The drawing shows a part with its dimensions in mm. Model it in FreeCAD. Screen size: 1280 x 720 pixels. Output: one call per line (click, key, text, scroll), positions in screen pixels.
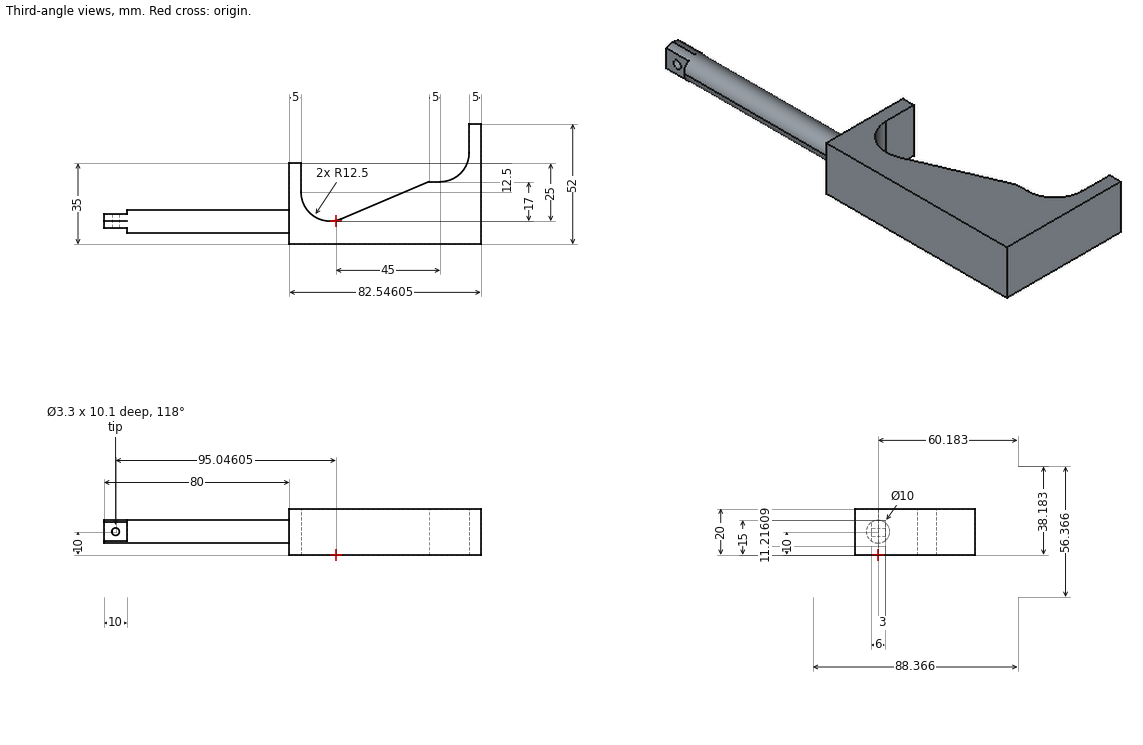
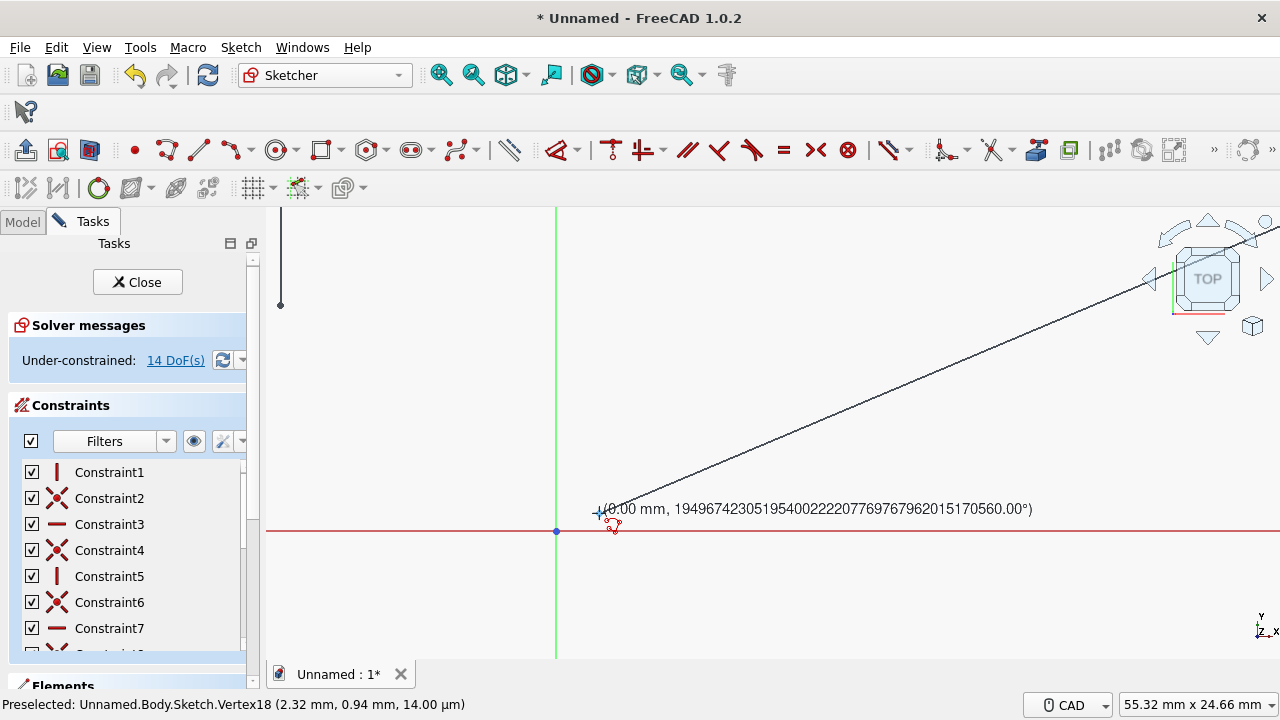
click(232, 150)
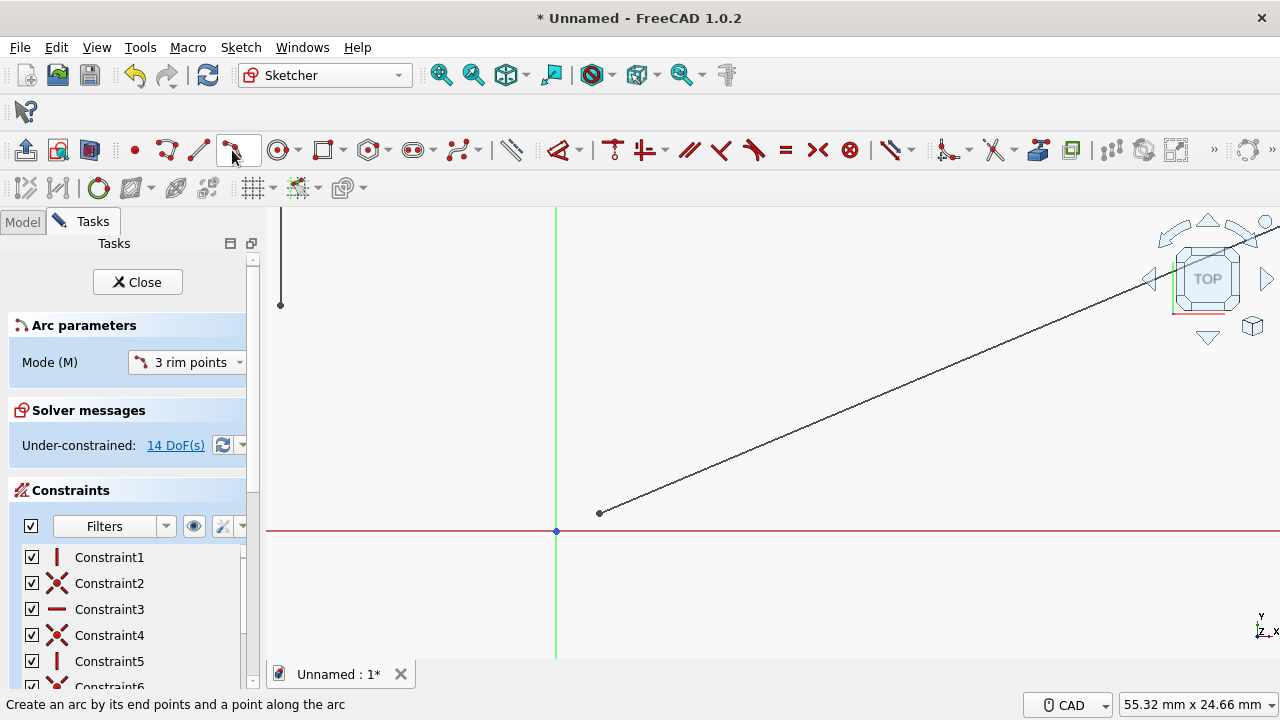
scroll(601, 517, down, 6)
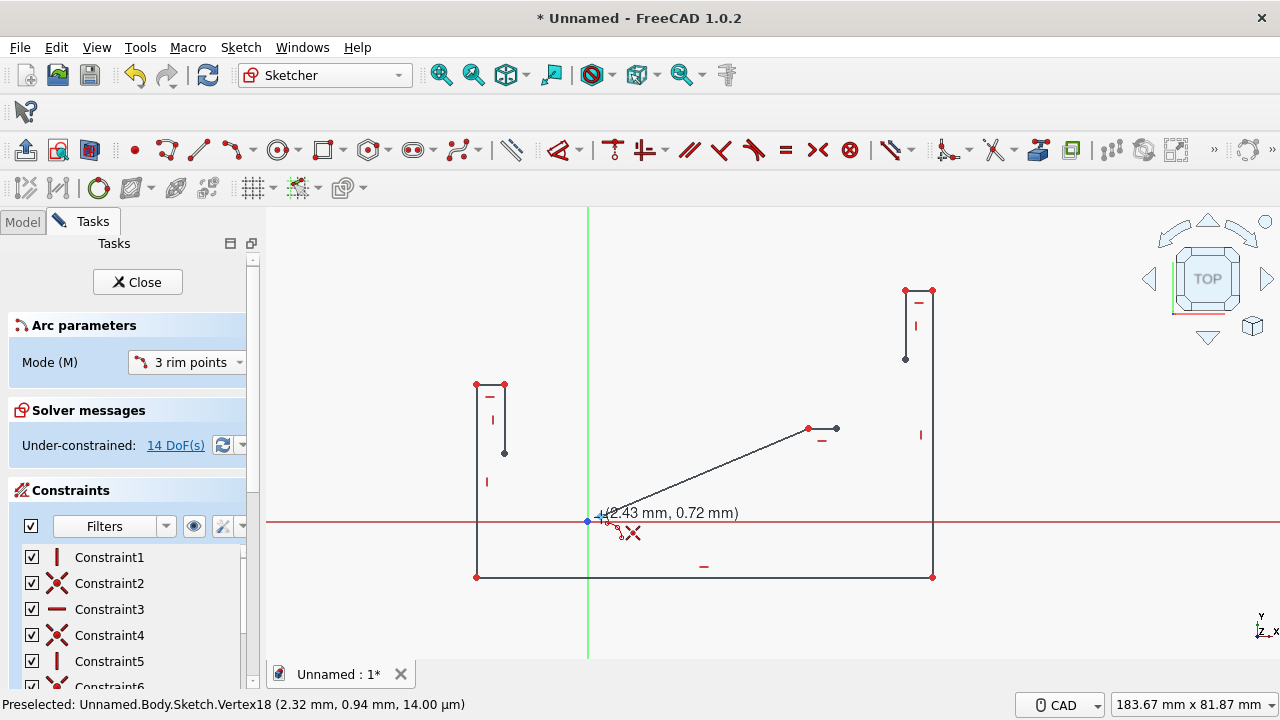
click(906, 360)
click(837, 429)
click(885, 408)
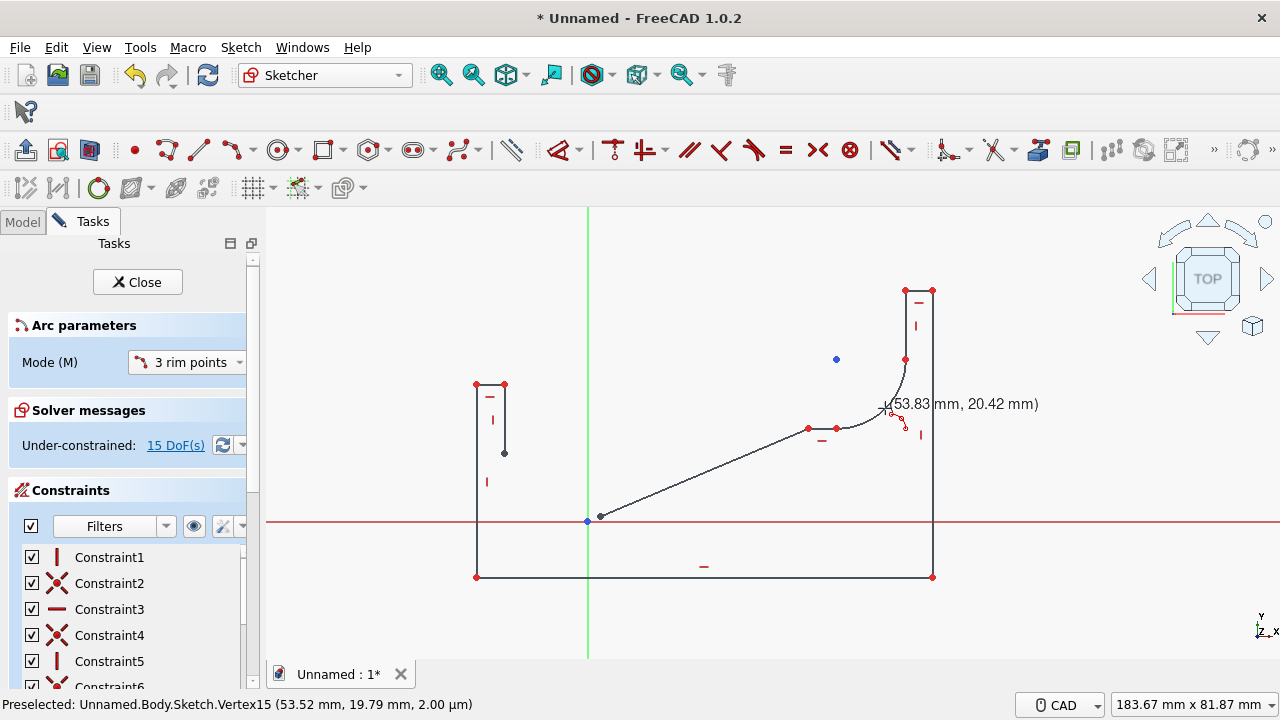
scroll(601, 516, up, 6)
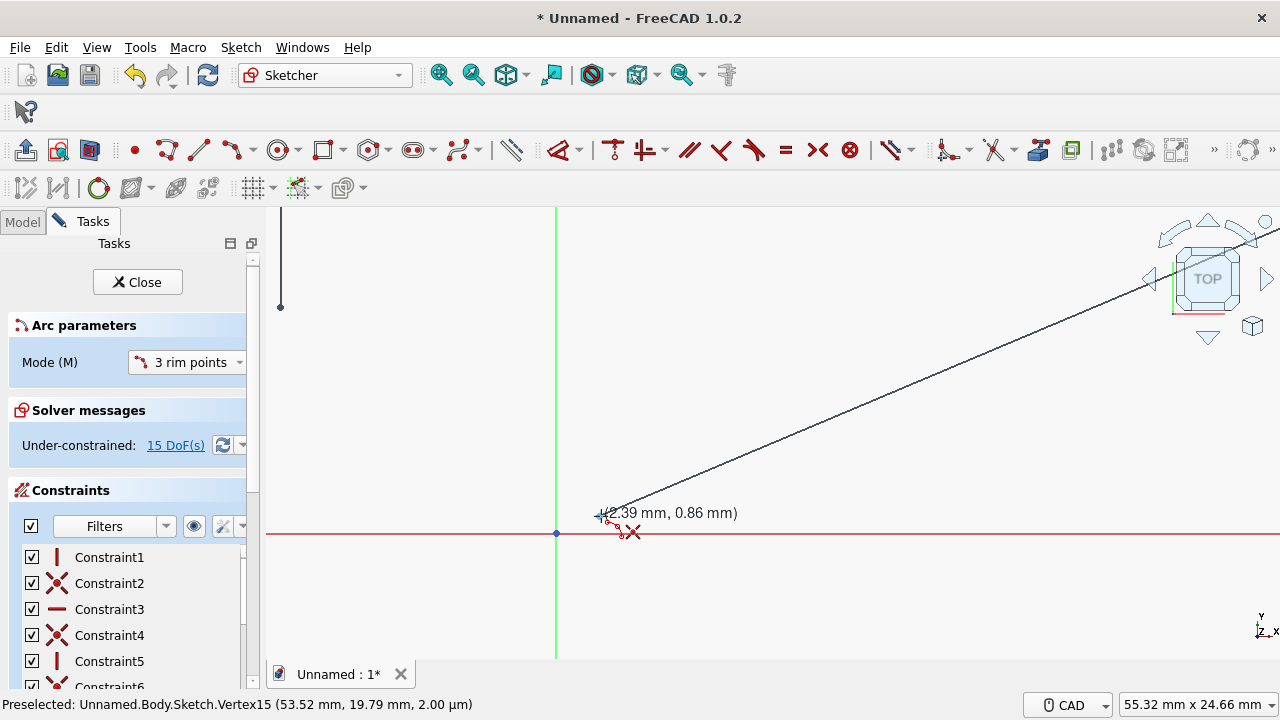
click(599, 516)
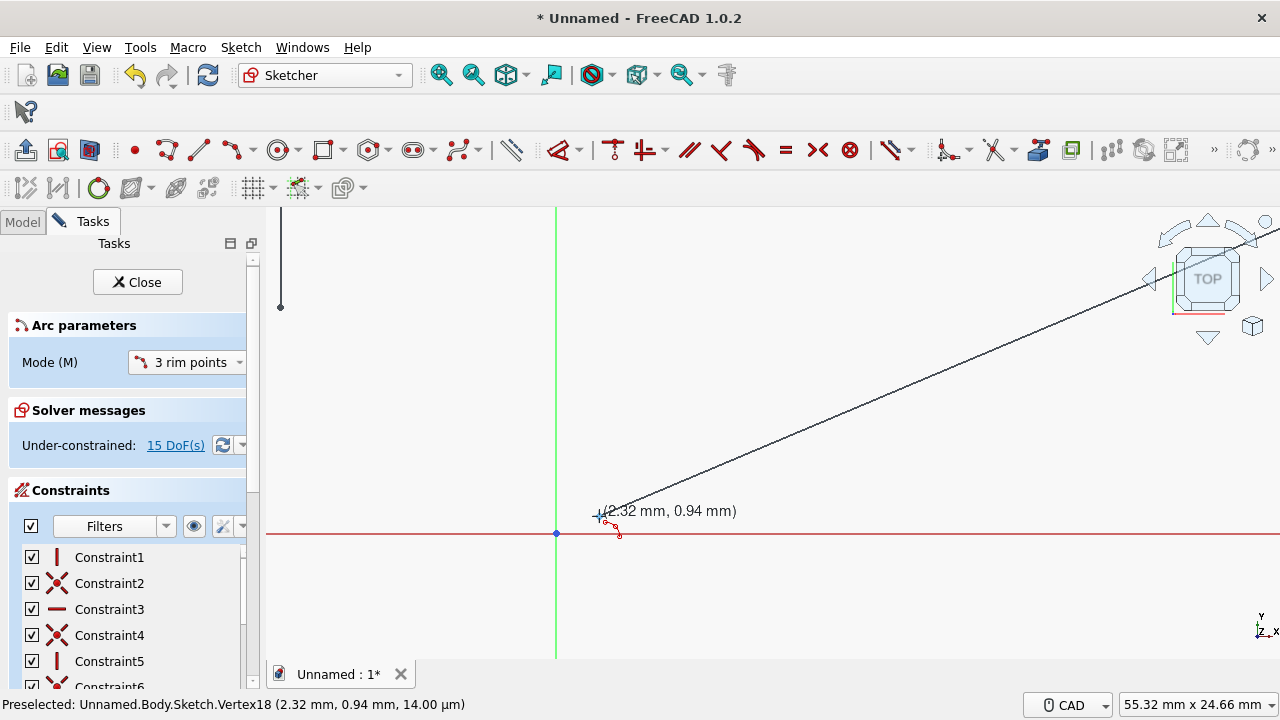
scroll(601, 516, down, 6)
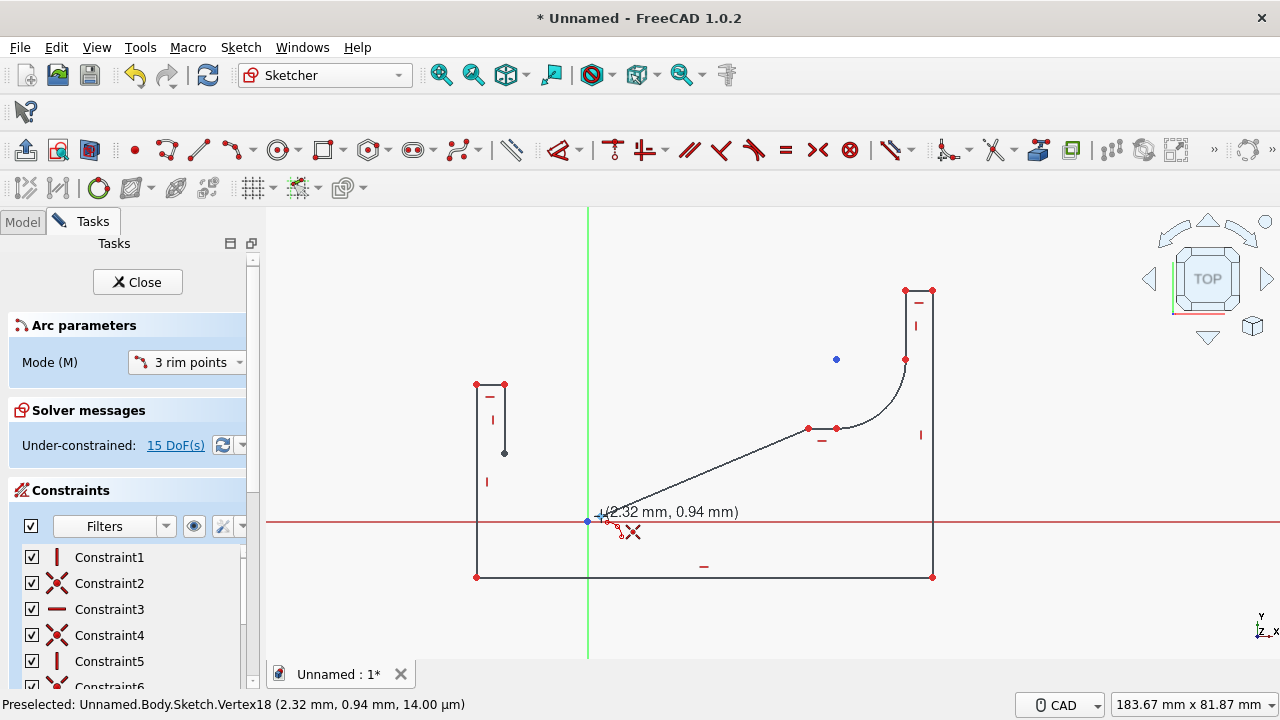
click(505, 454)
click(525, 502)
key(Escape)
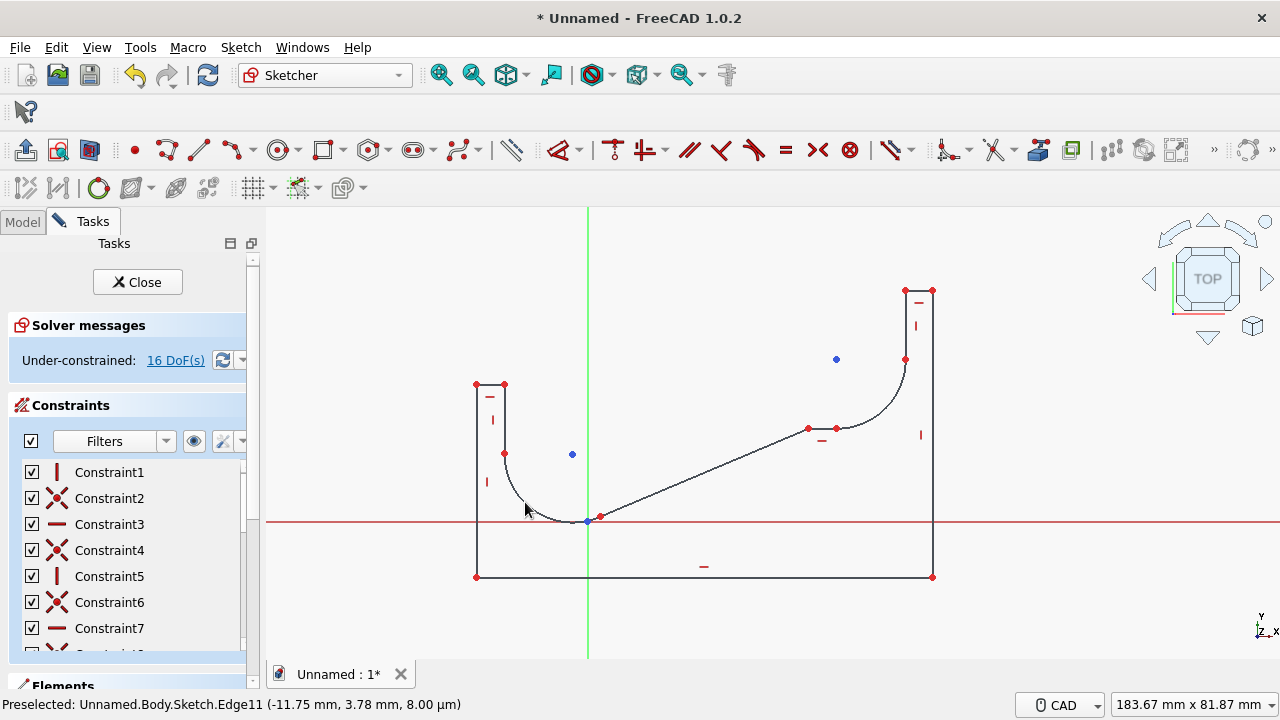
click(505, 433)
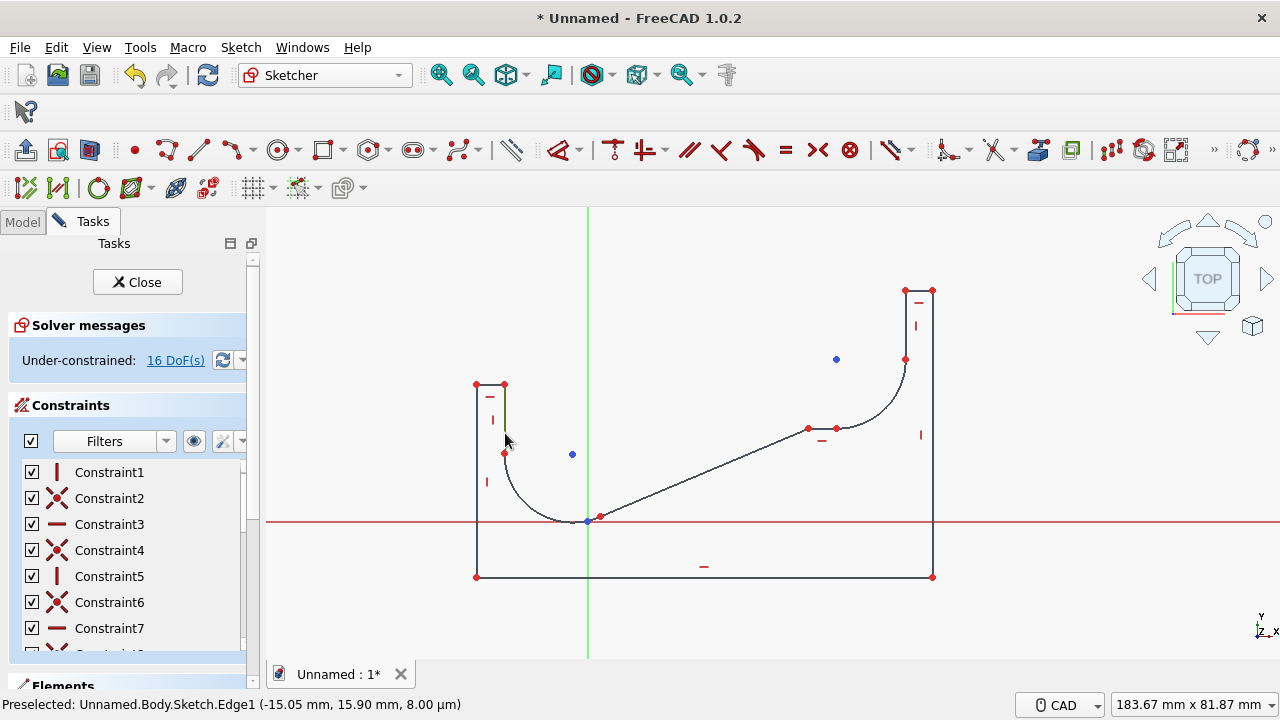
click(516, 492)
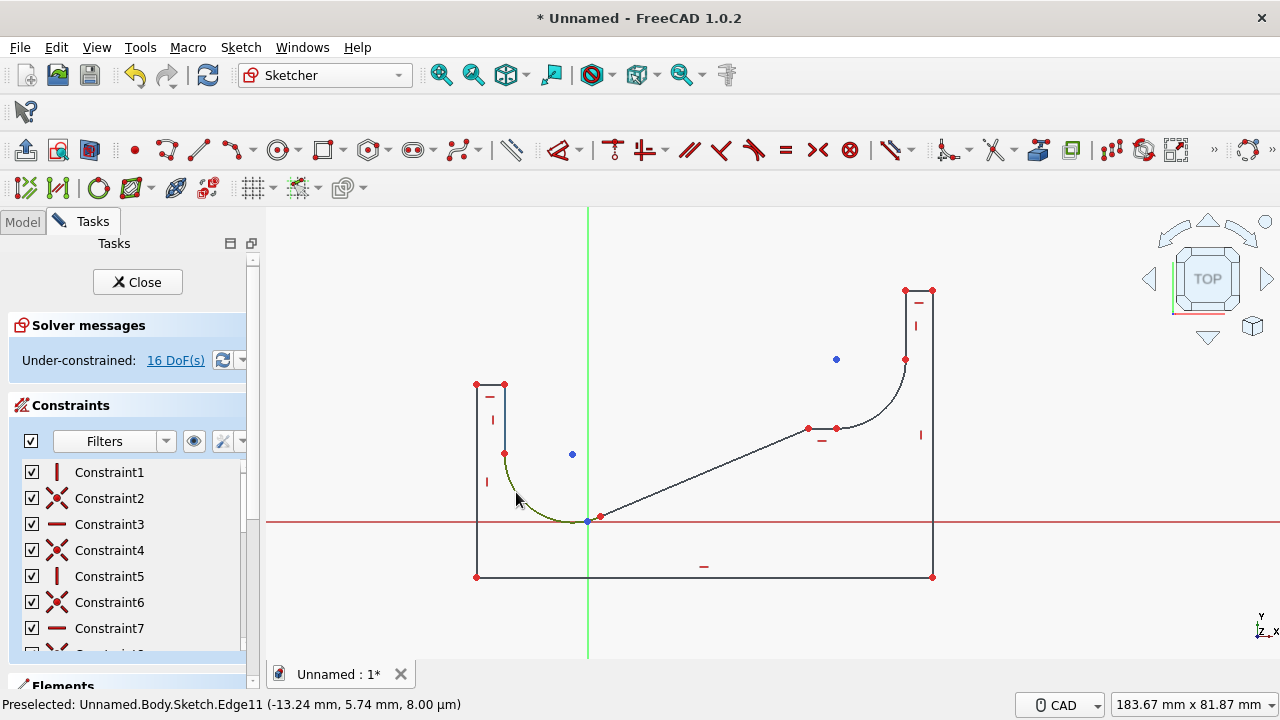
click(754, 150)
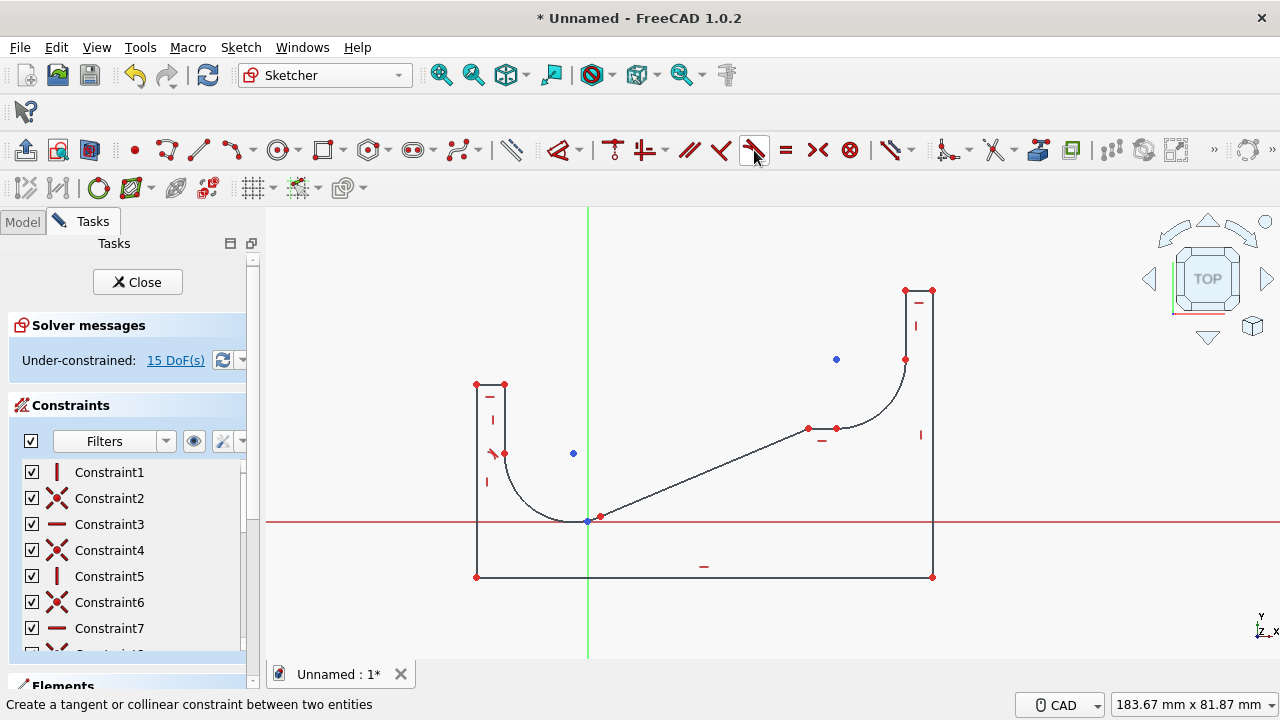
click(906, 311)